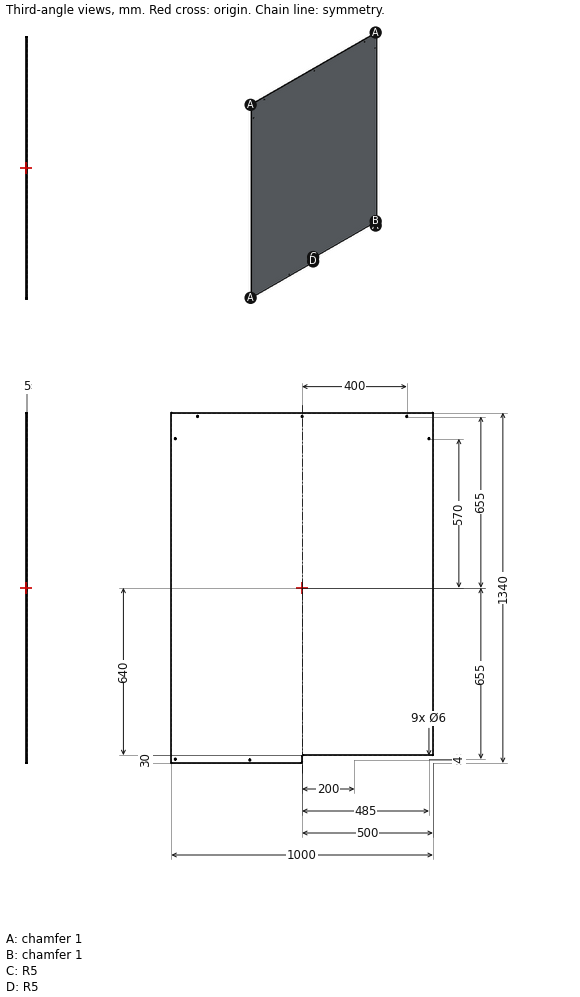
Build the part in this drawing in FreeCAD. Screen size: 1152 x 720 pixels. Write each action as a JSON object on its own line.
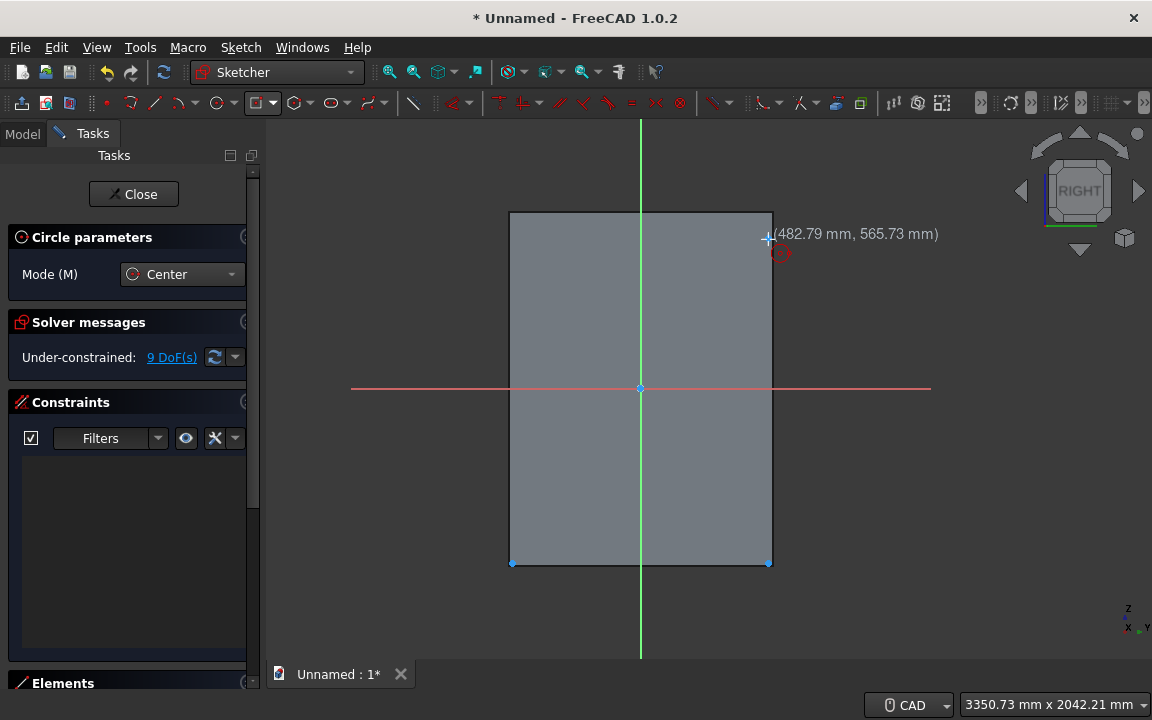
{"action": "scroll", "coordinate": [747, 216], "scroll_direction": "up", "scroll_amount": 17}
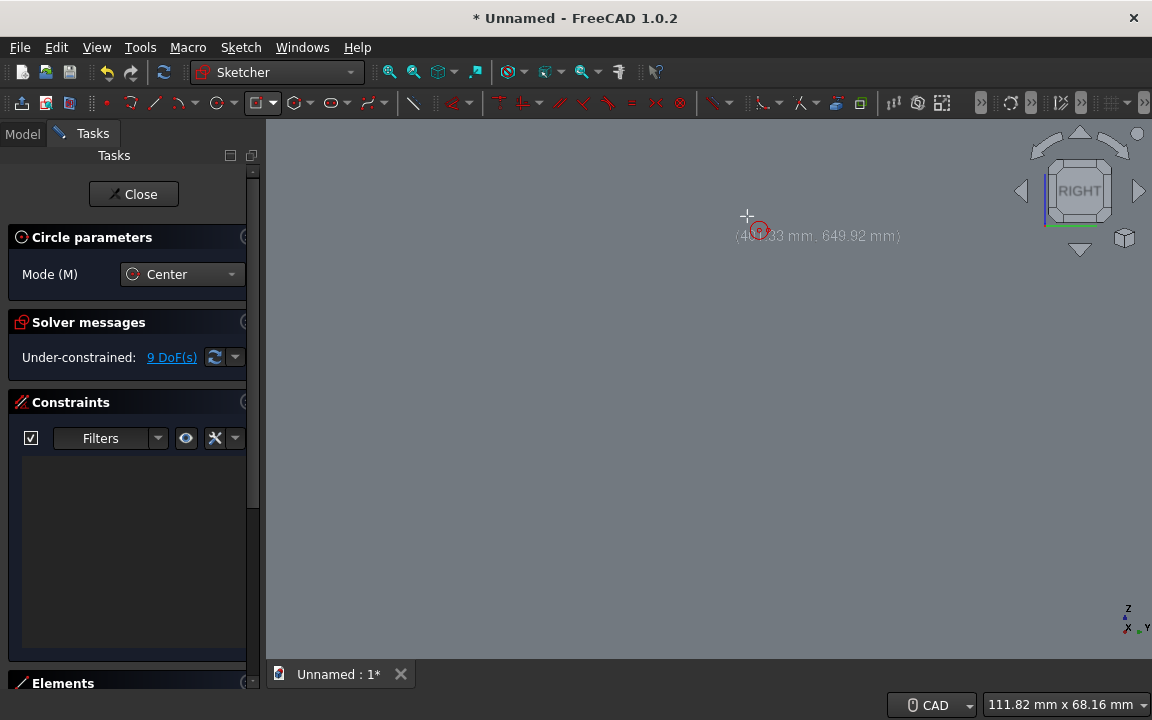
{"action": "scroll", "coordinate": [772, 176], "scroll_direction": "down", "scroll_amount": 16}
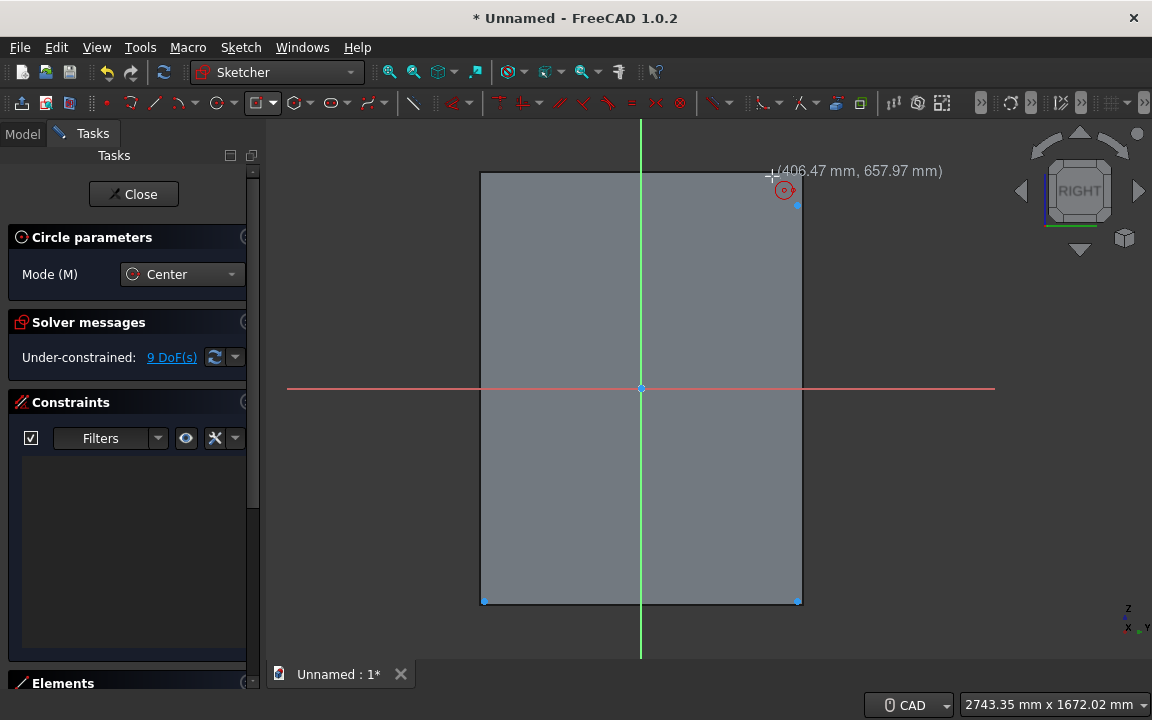
{"action": "left_click", "coordinate": [770, 177]}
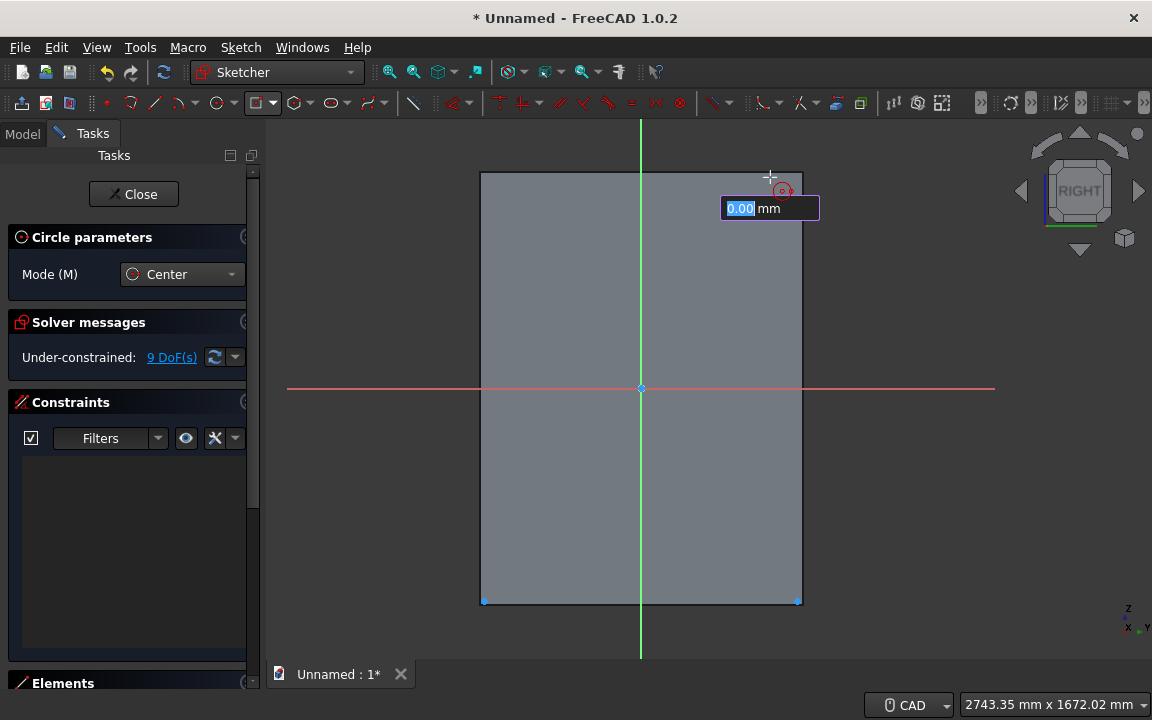
{"action": "scroll", "coordinate": [771, 176], "scroll_direction": "up", "scroll_amount": 14}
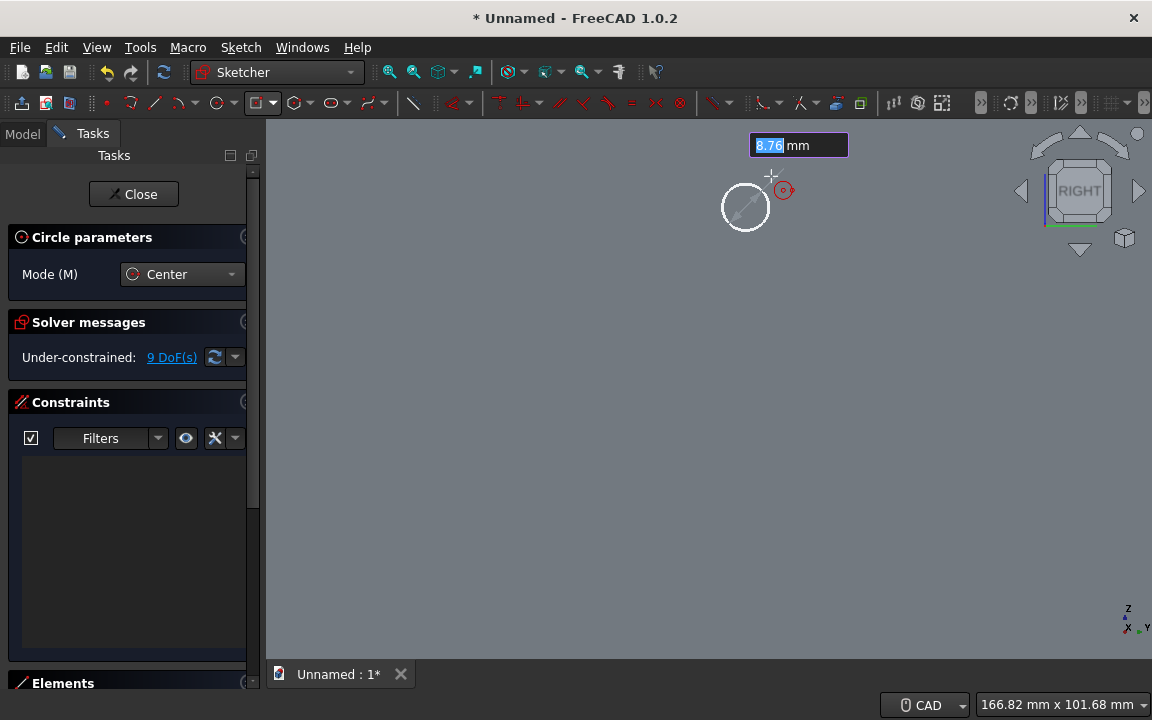
{"action": "left_click", "coordinate": [765, 181]}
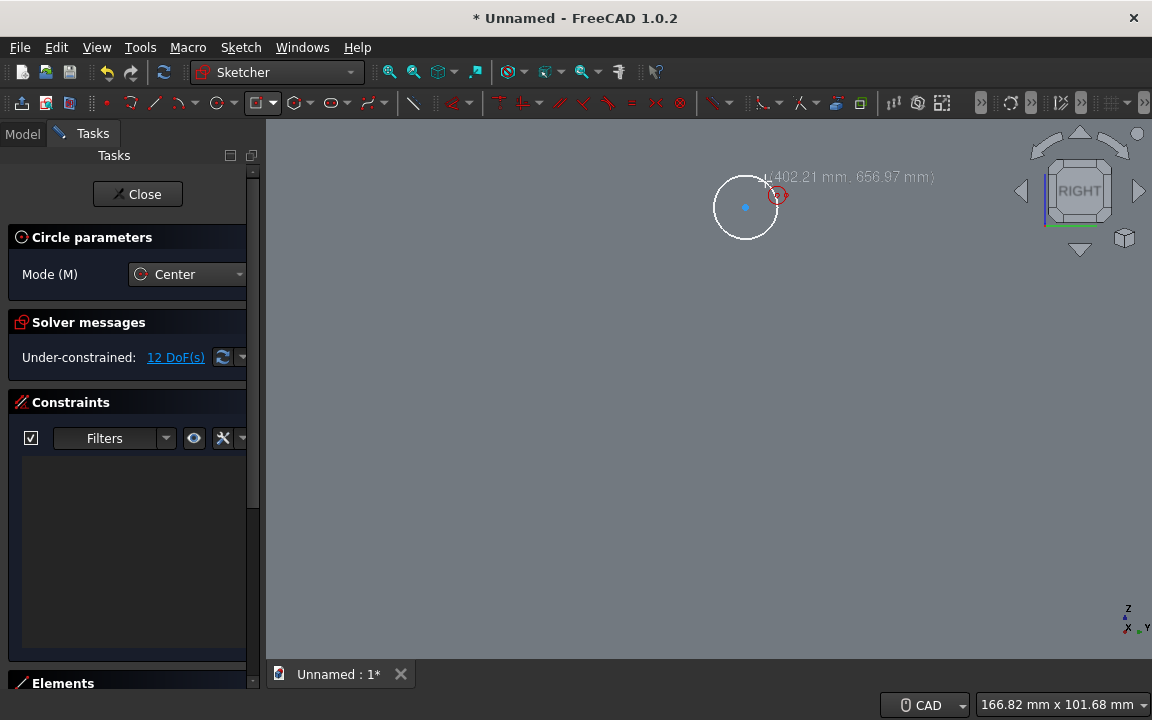
{"action": "scroll", "coordinate": [746, 216], "scroll_direction": "down", "scroll_amount": 15}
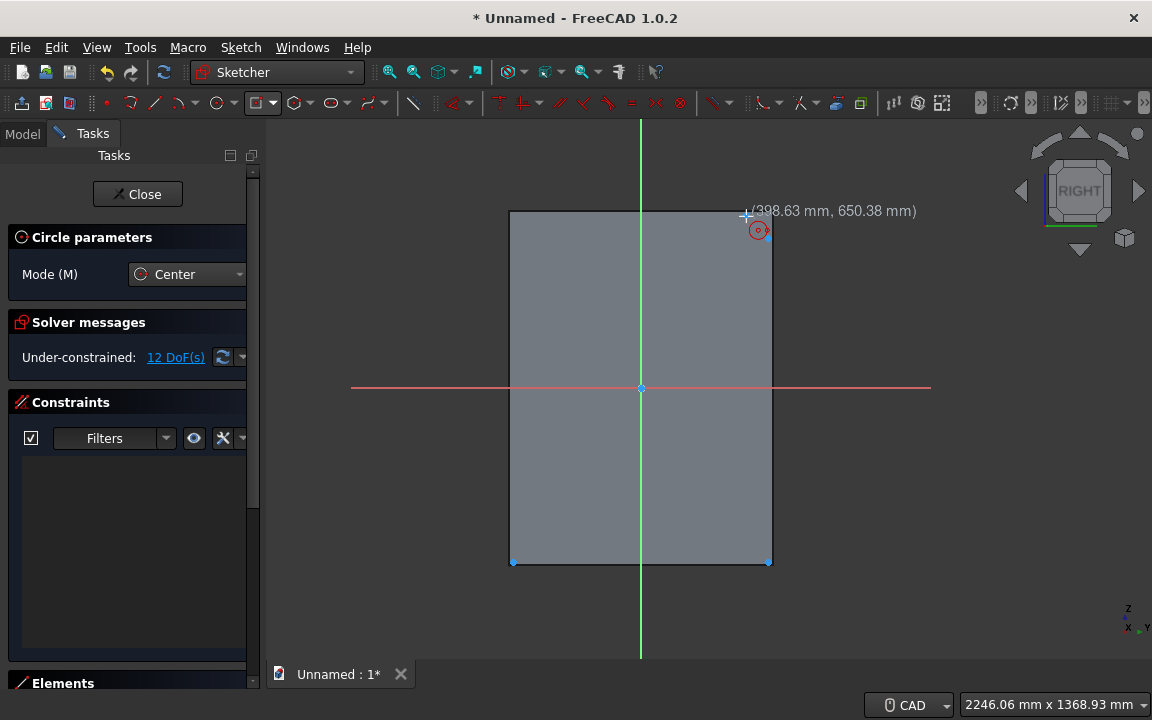
{"action": "scroll", "coordinate": [535, 215], "scroll_direction": "up", "scroll_amount": 17}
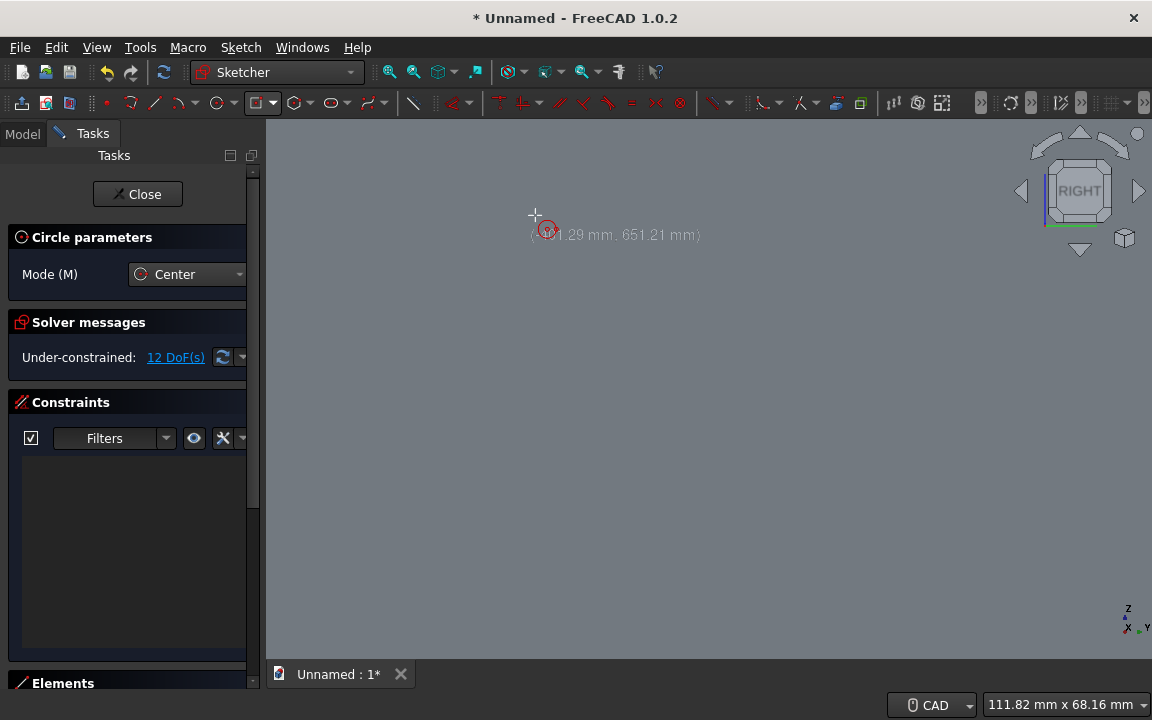
{"action": "scroll", "coordinate": [510, 175], "scroll_direction": "down", "scroll_amount": 16}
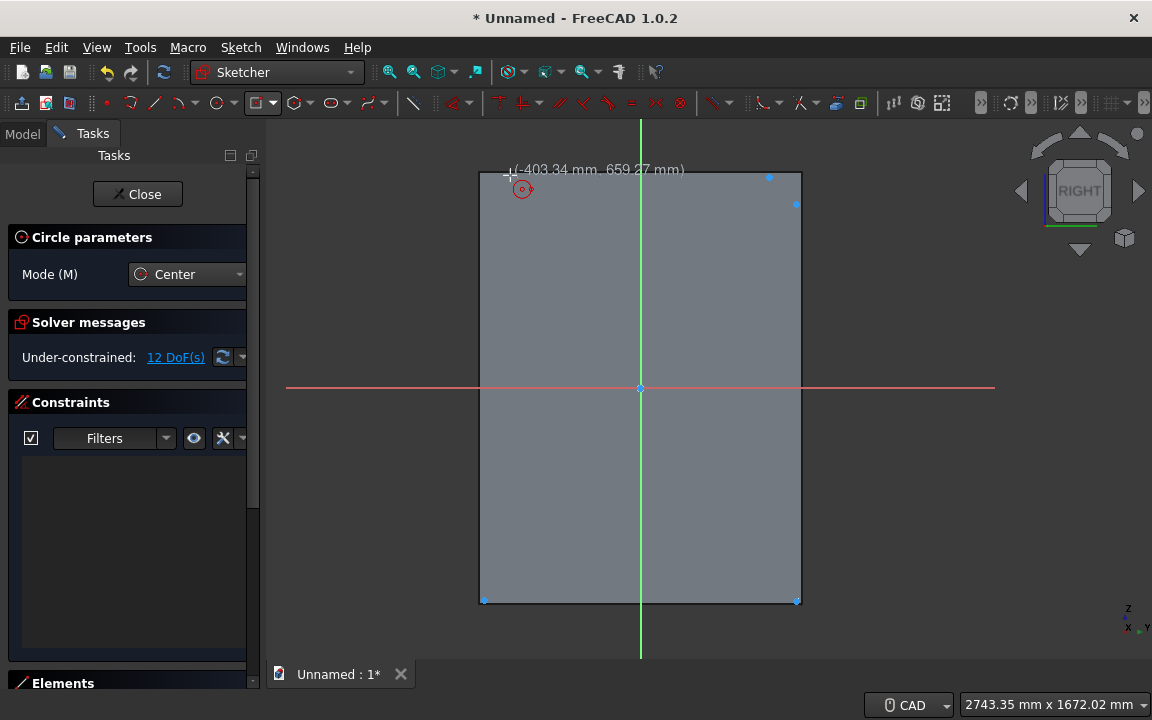
{"action": "left_click", "coordinate": [511, 177]}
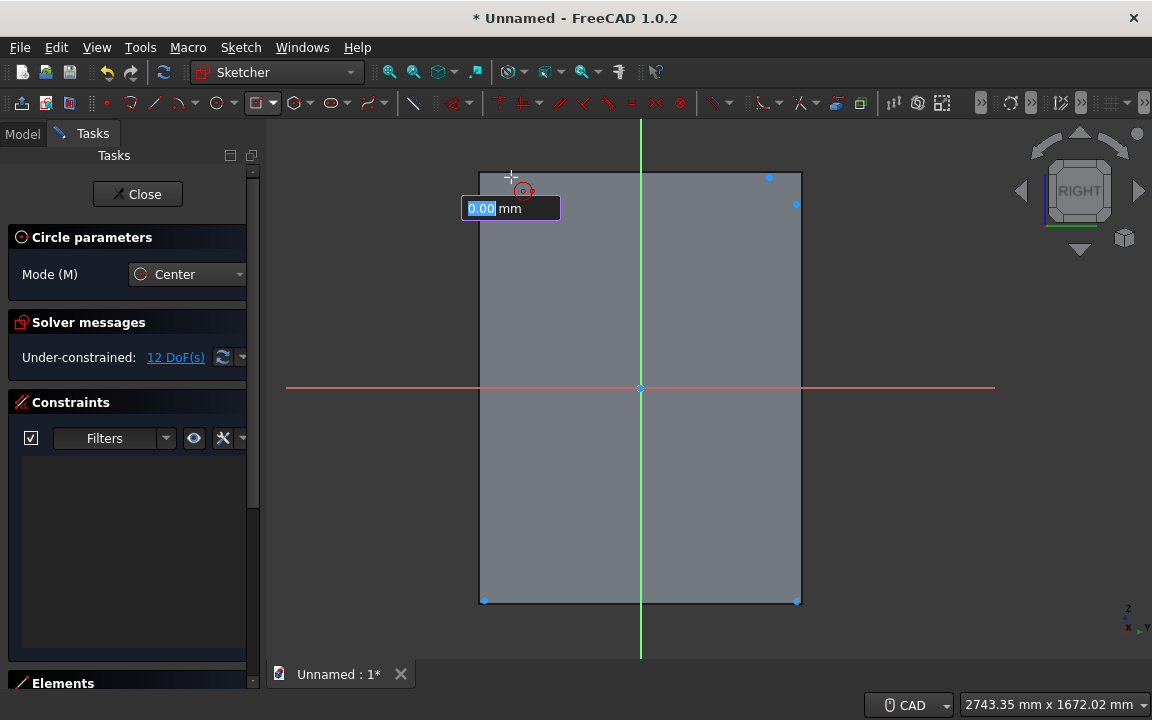
{"action": "scroll", "coordinate": [512, 176], "scroll_direction": "up", "scroll_amount": 14}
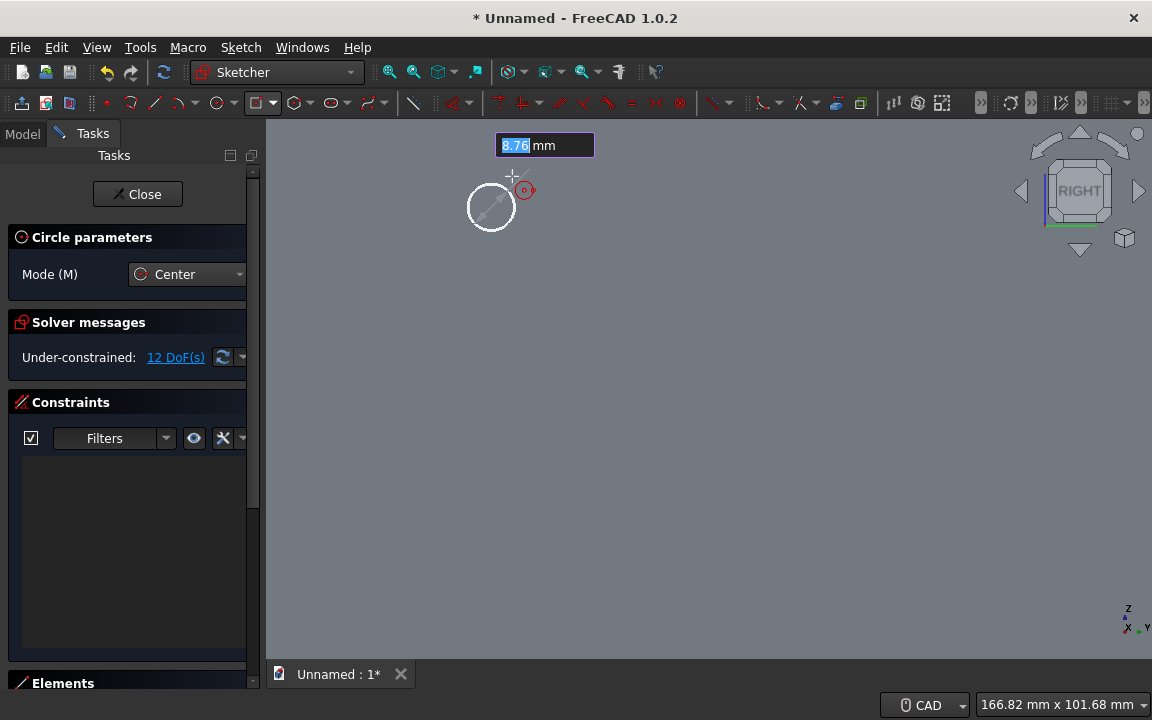
{"action": "left_click", "coordinate": [508, 172]}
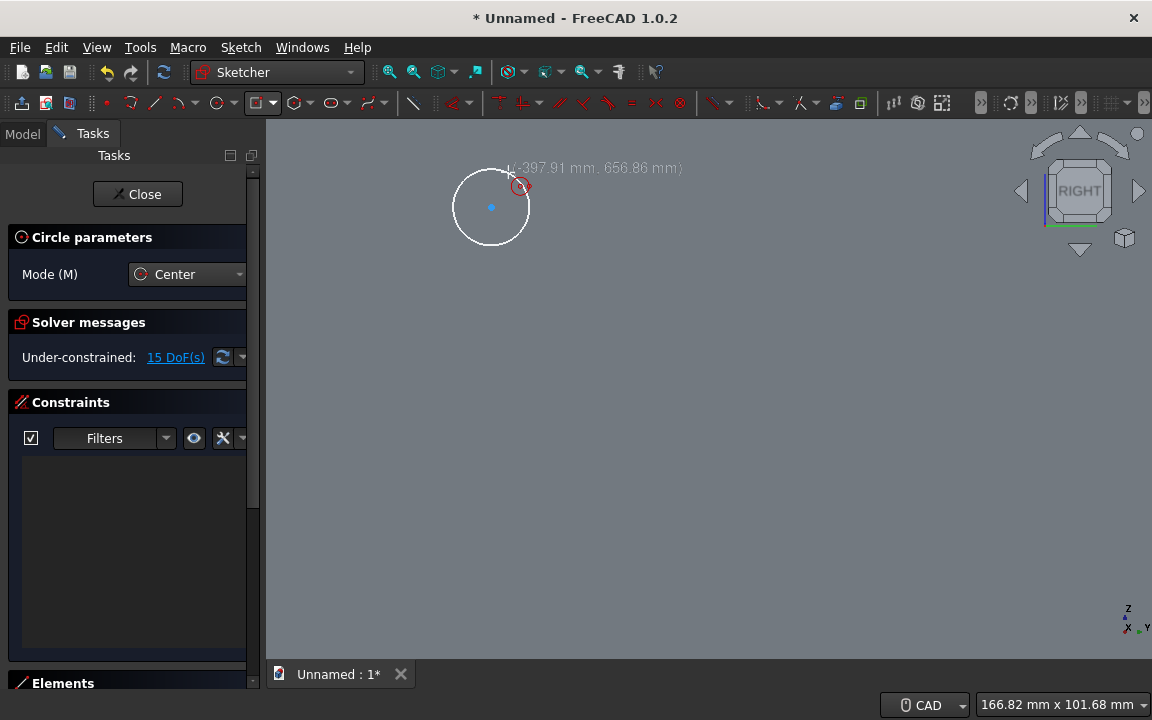
{"action": "scroll", "coordinate": [537, 217], "scroll_direction": "down", "scroll_amount": 15}